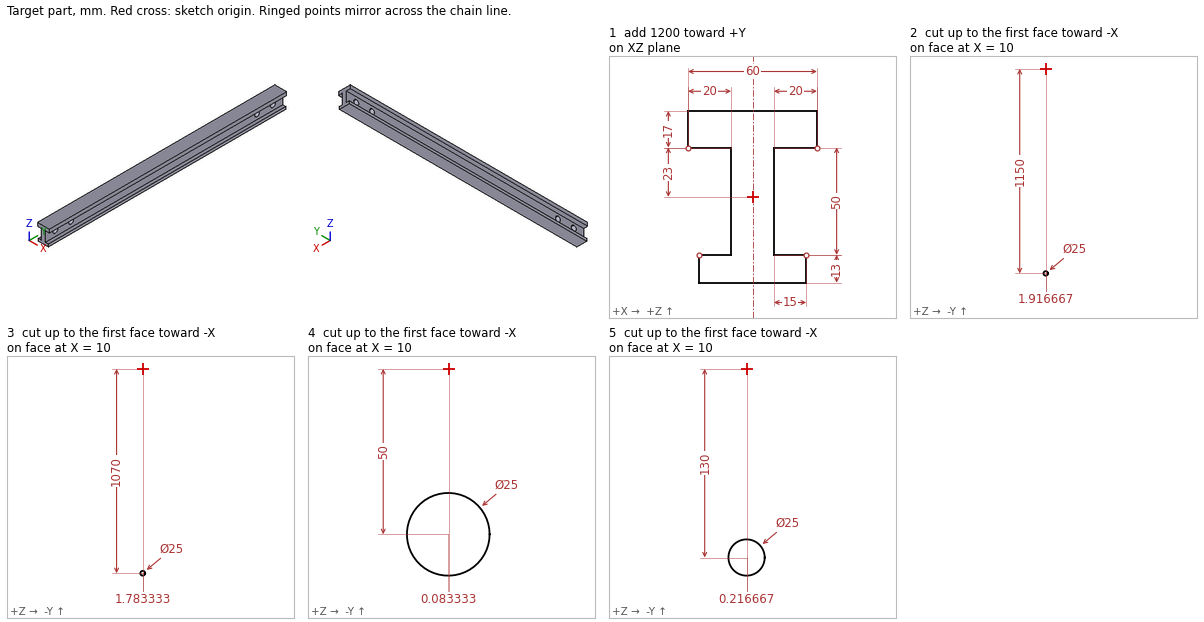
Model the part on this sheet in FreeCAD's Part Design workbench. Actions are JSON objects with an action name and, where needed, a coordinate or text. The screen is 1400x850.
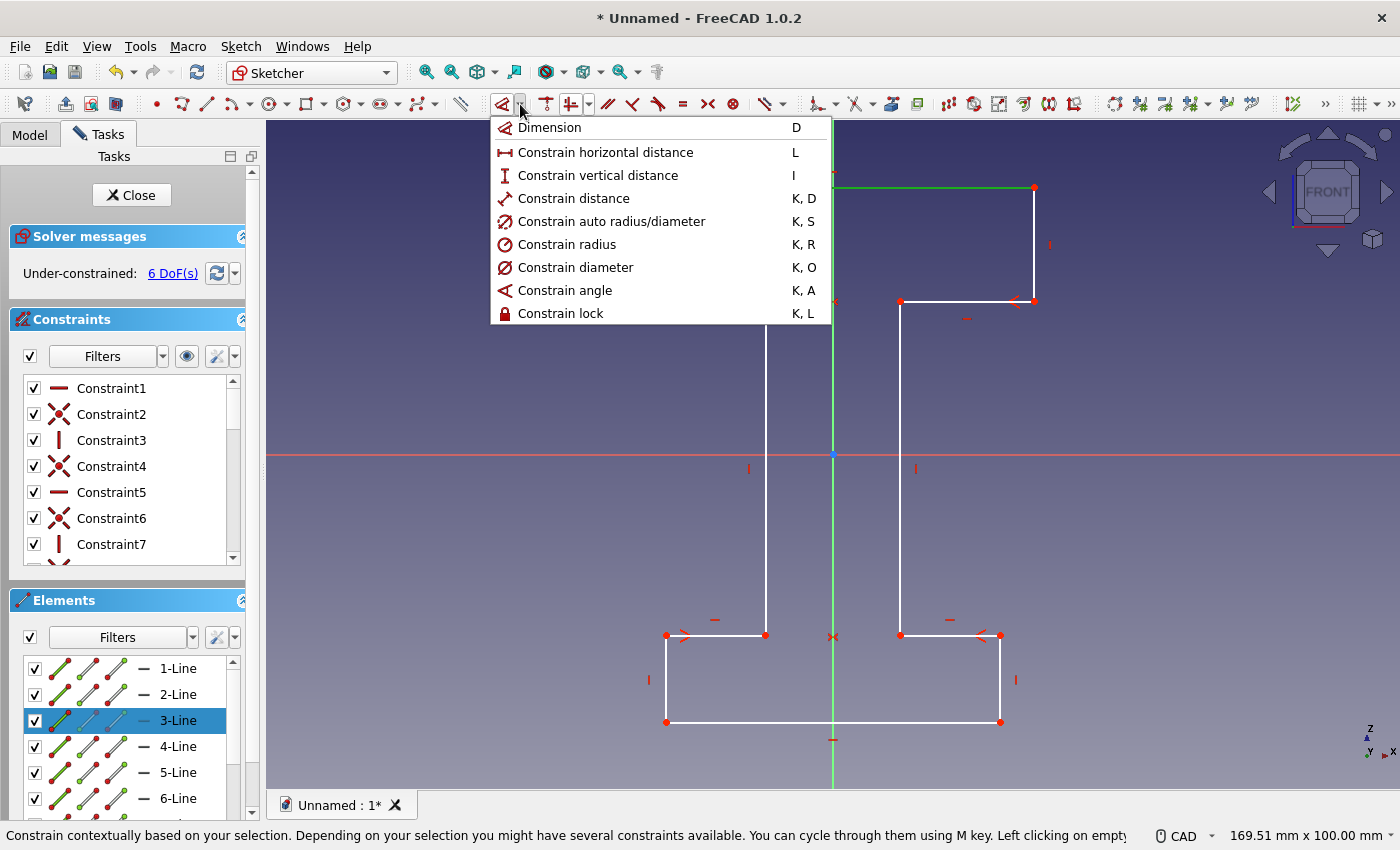
{"action": "left_click", "coordinate": [661, 152]}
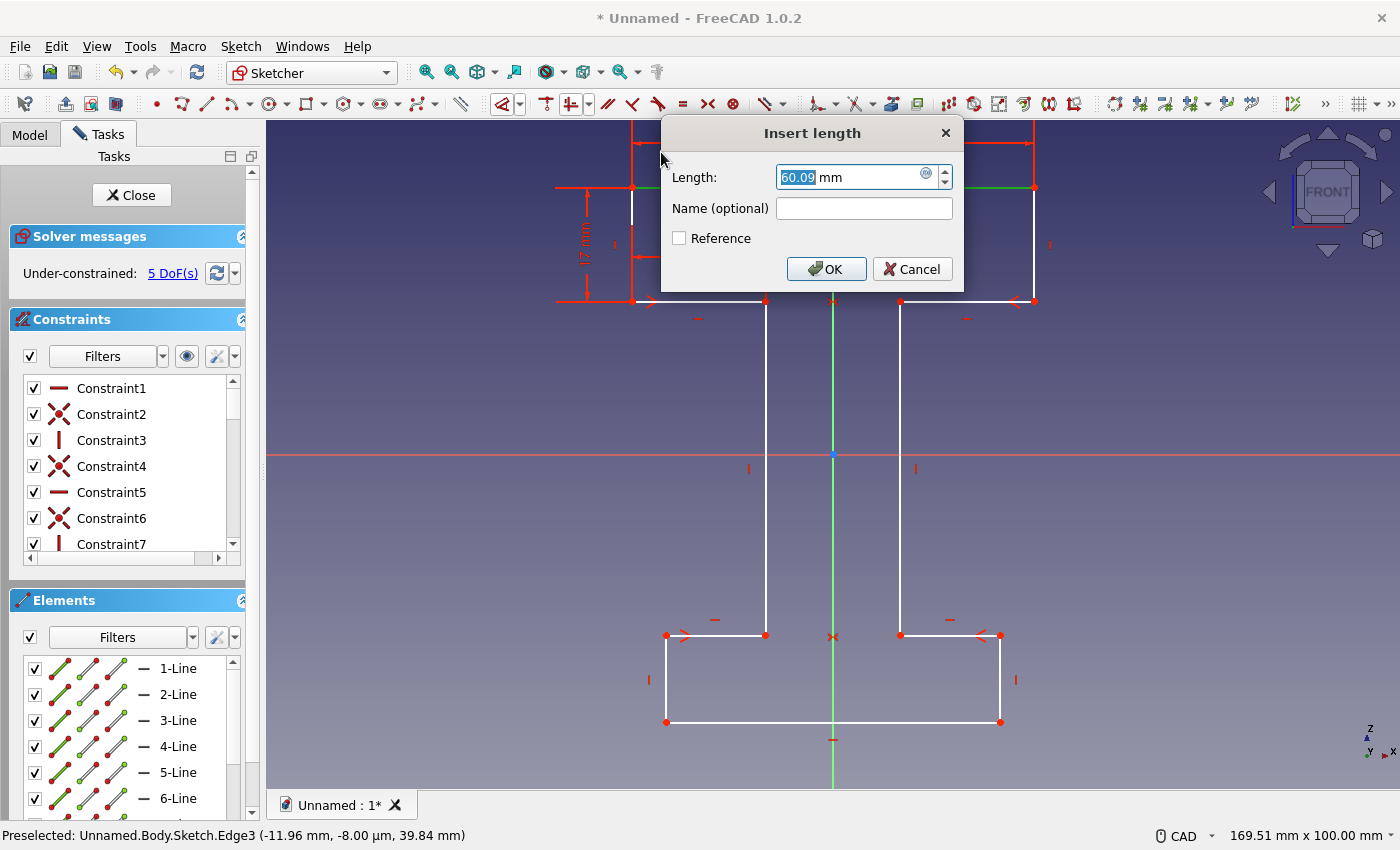
{"action": "type", "text": "60"}
{"action": "key", "text": "Return"}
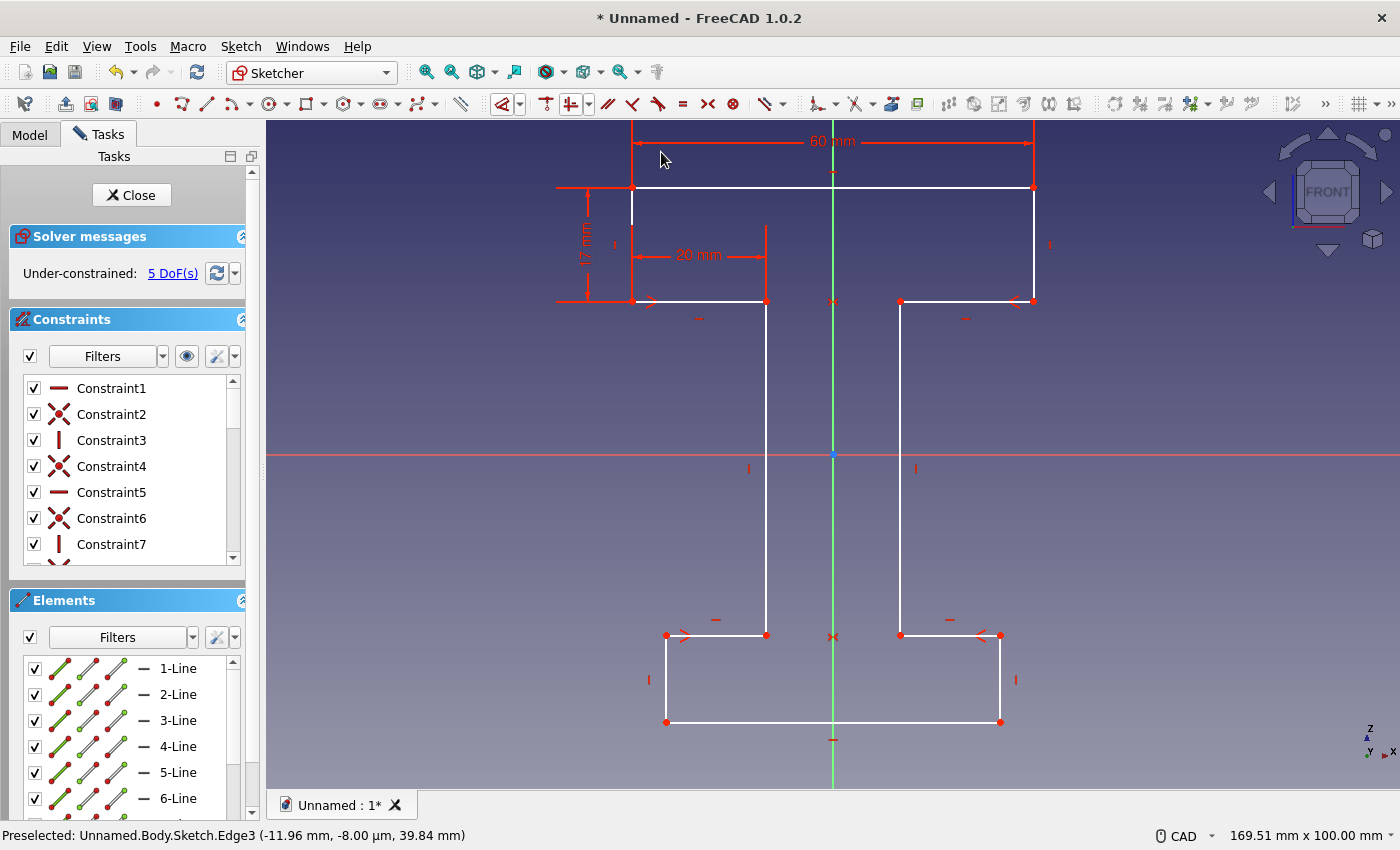
{"action": "left_click", "coordinate": [994, 302]}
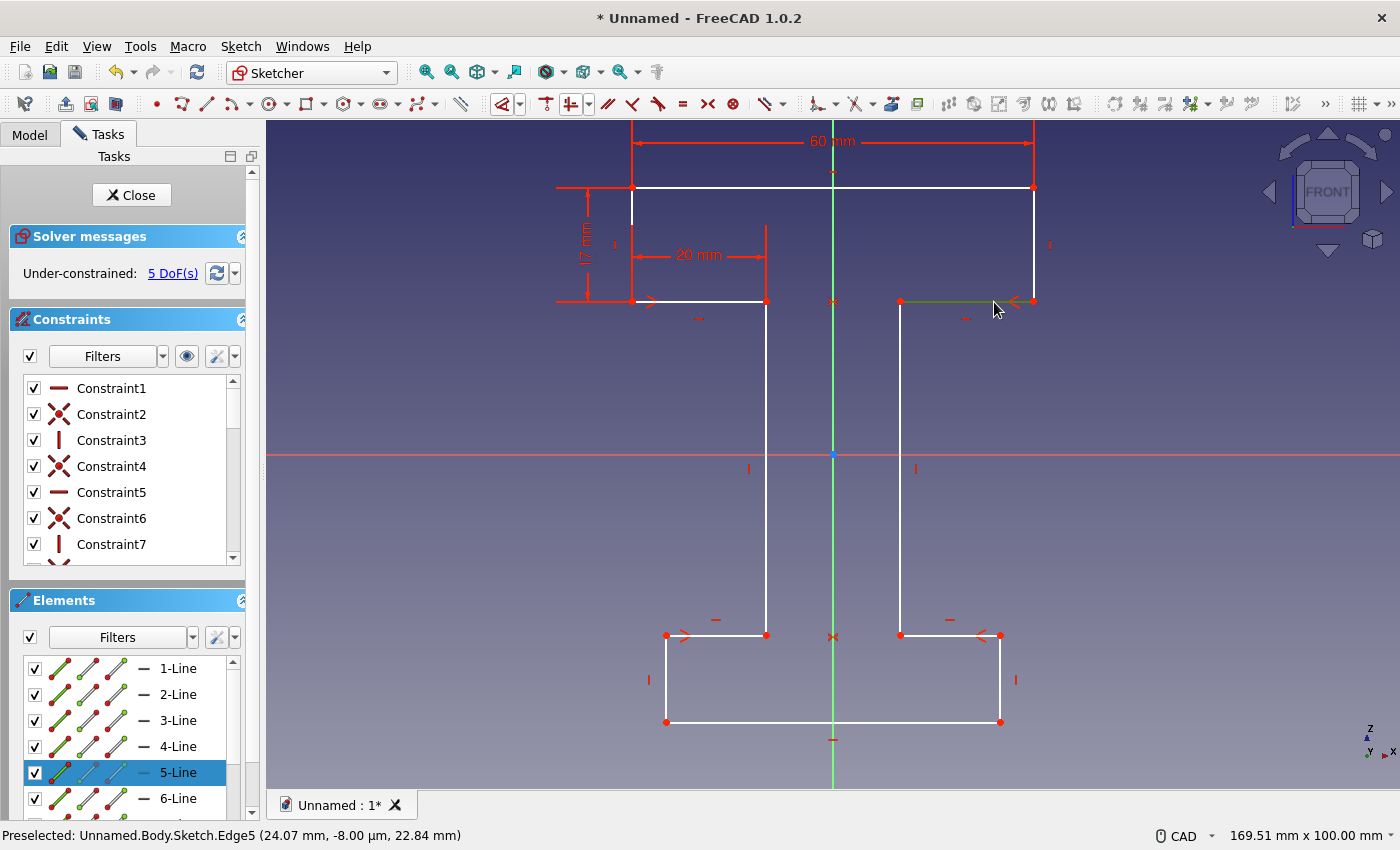
{"action": "left_click", "coordinate": [520, 104]}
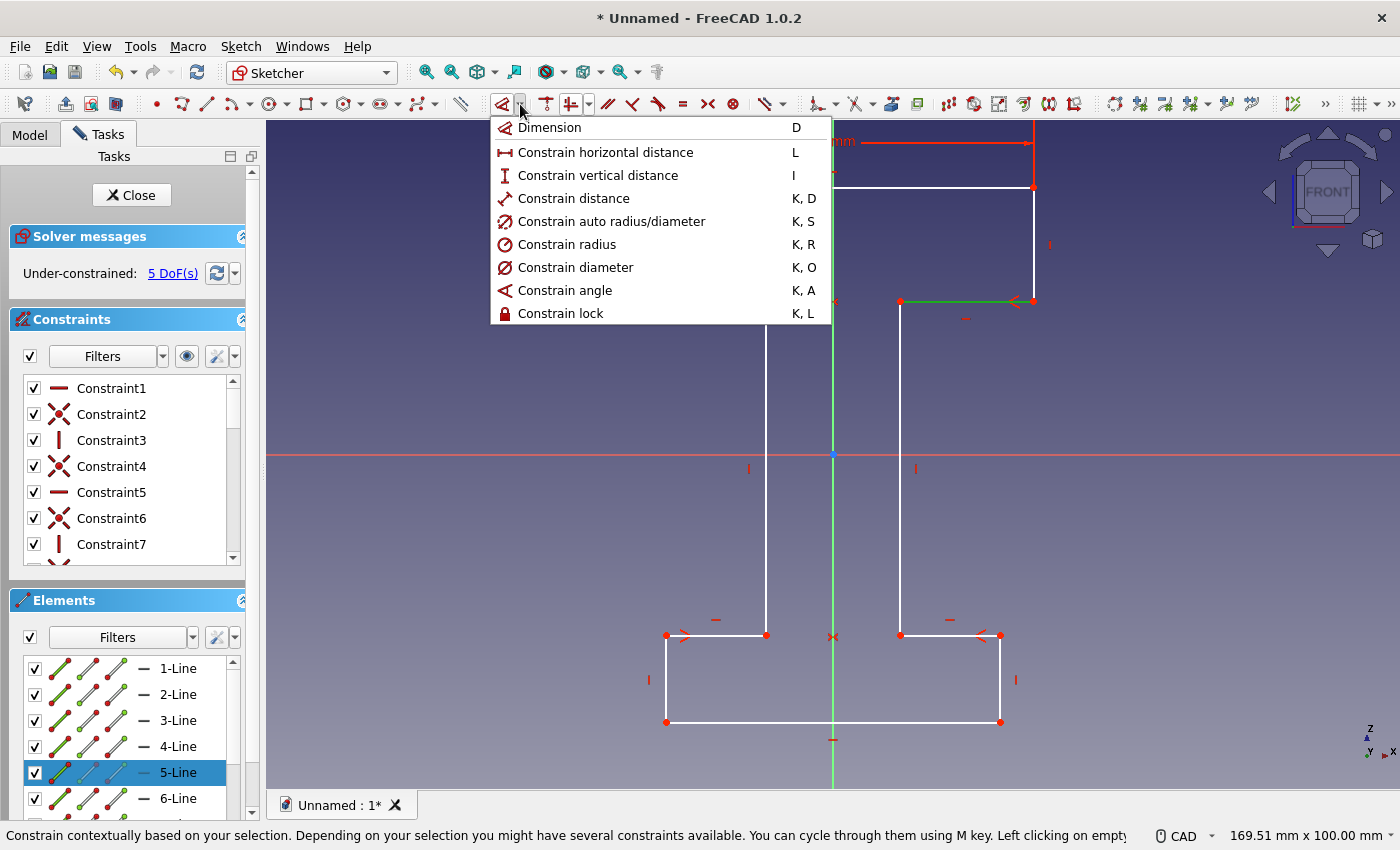
{"action": "left_click", "coordinate": [661, 152]}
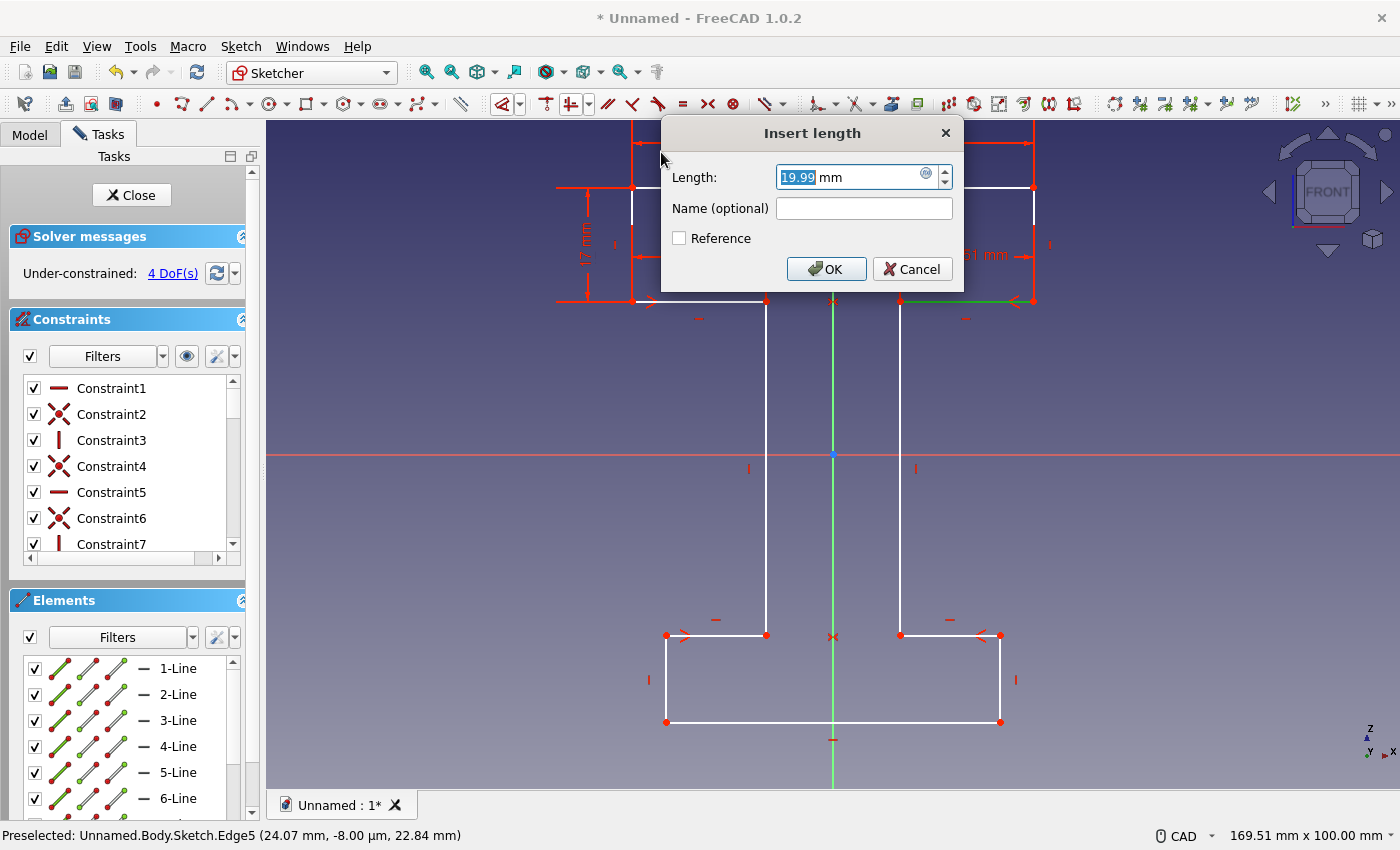
{"action": "type", "text": "20"}
{"action": "key", "text": "Return"}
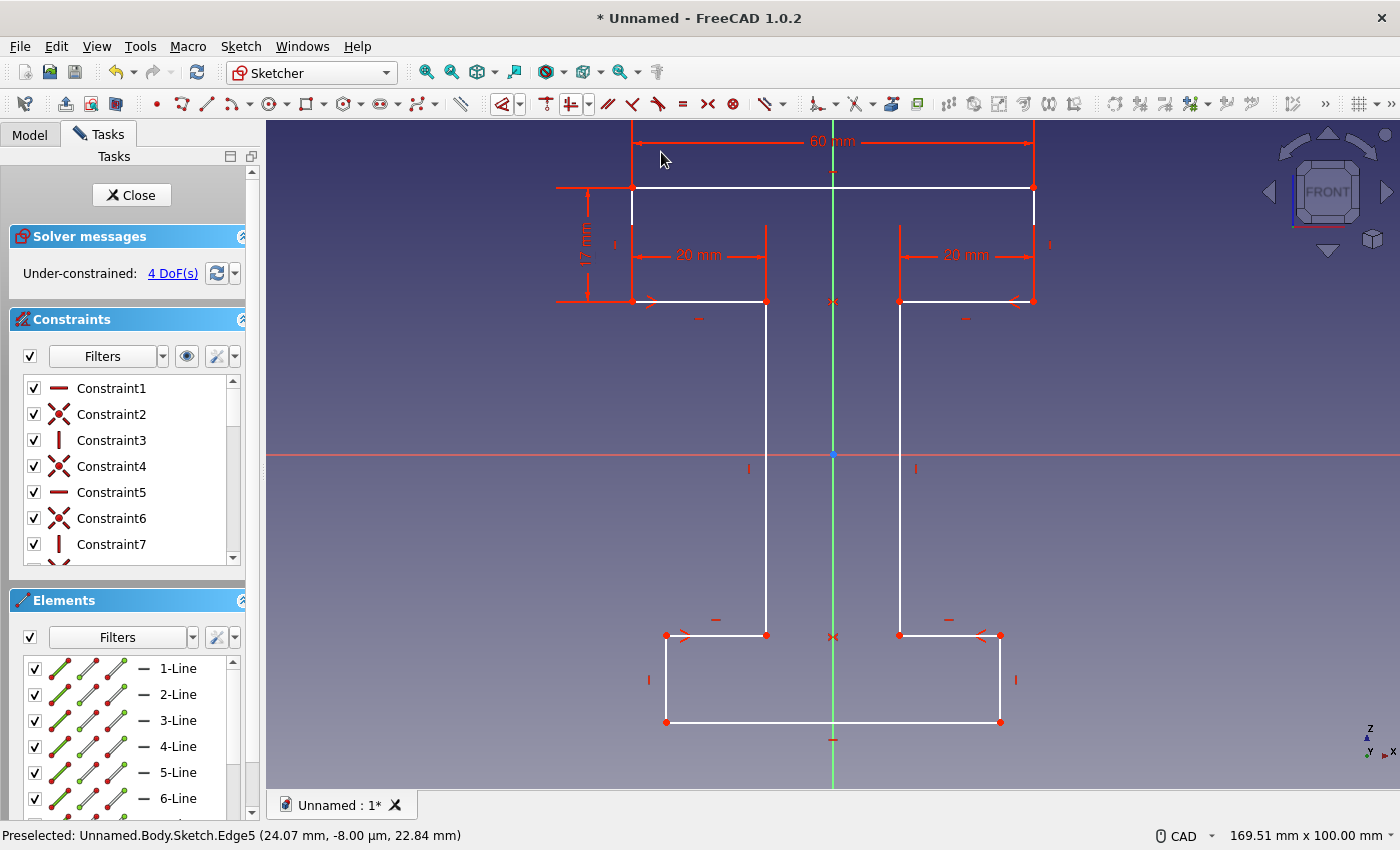
{"action": "left_click", "coordinate": [900, 402]}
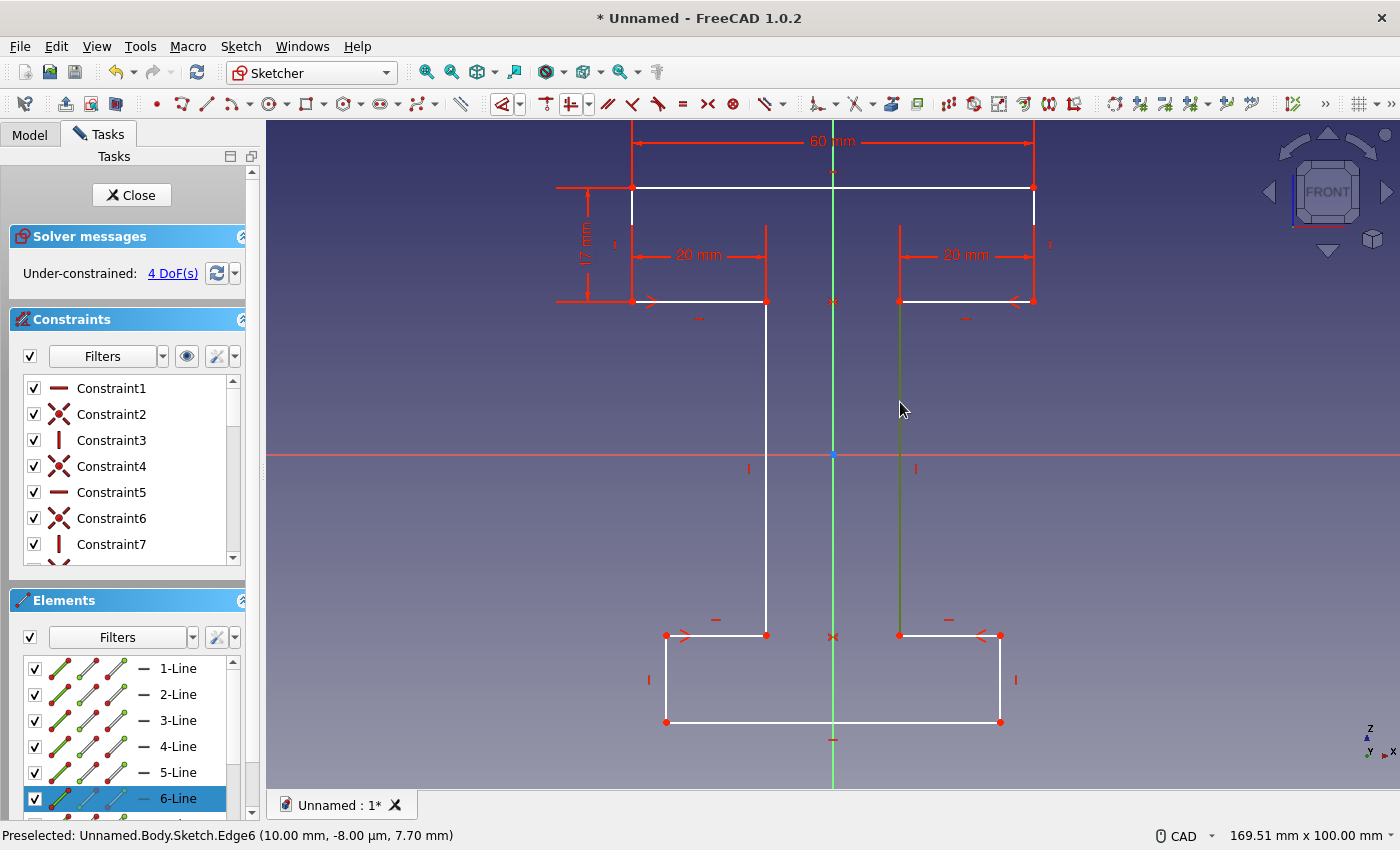
{"action": "key", "text": "i"}